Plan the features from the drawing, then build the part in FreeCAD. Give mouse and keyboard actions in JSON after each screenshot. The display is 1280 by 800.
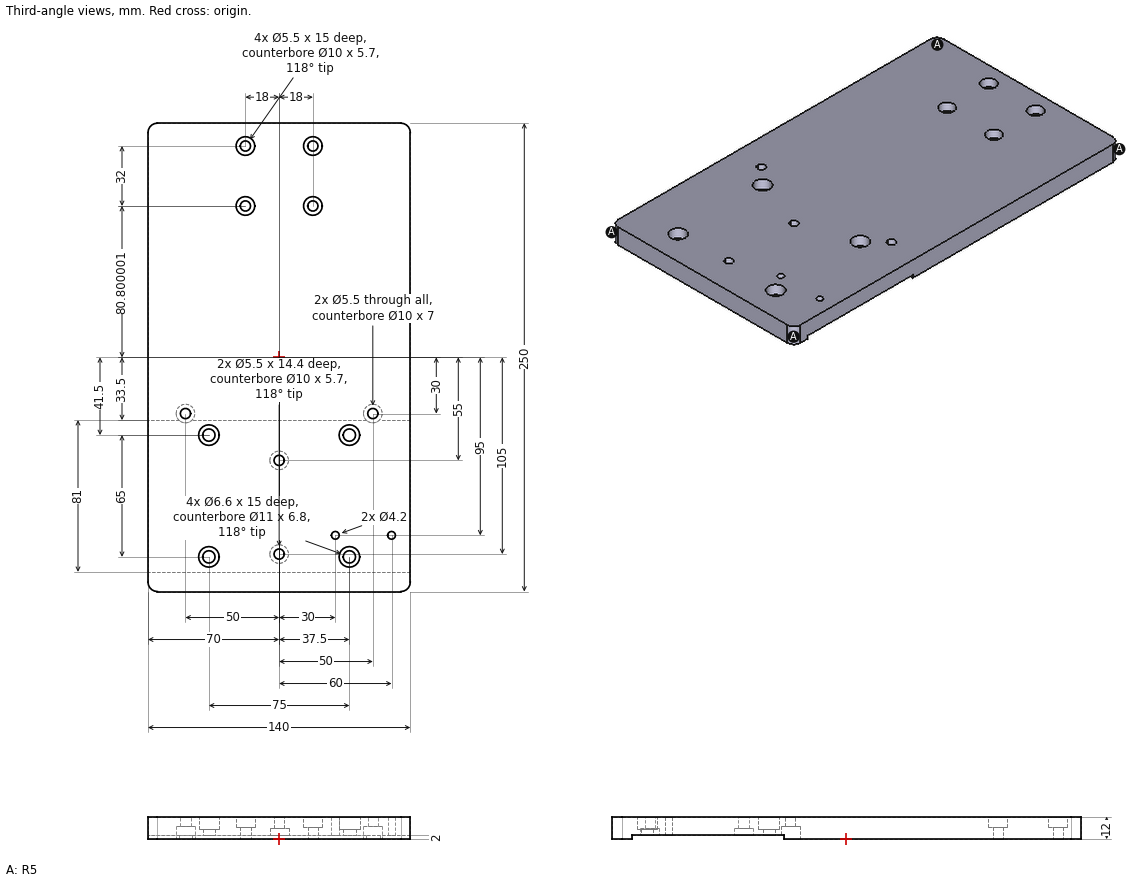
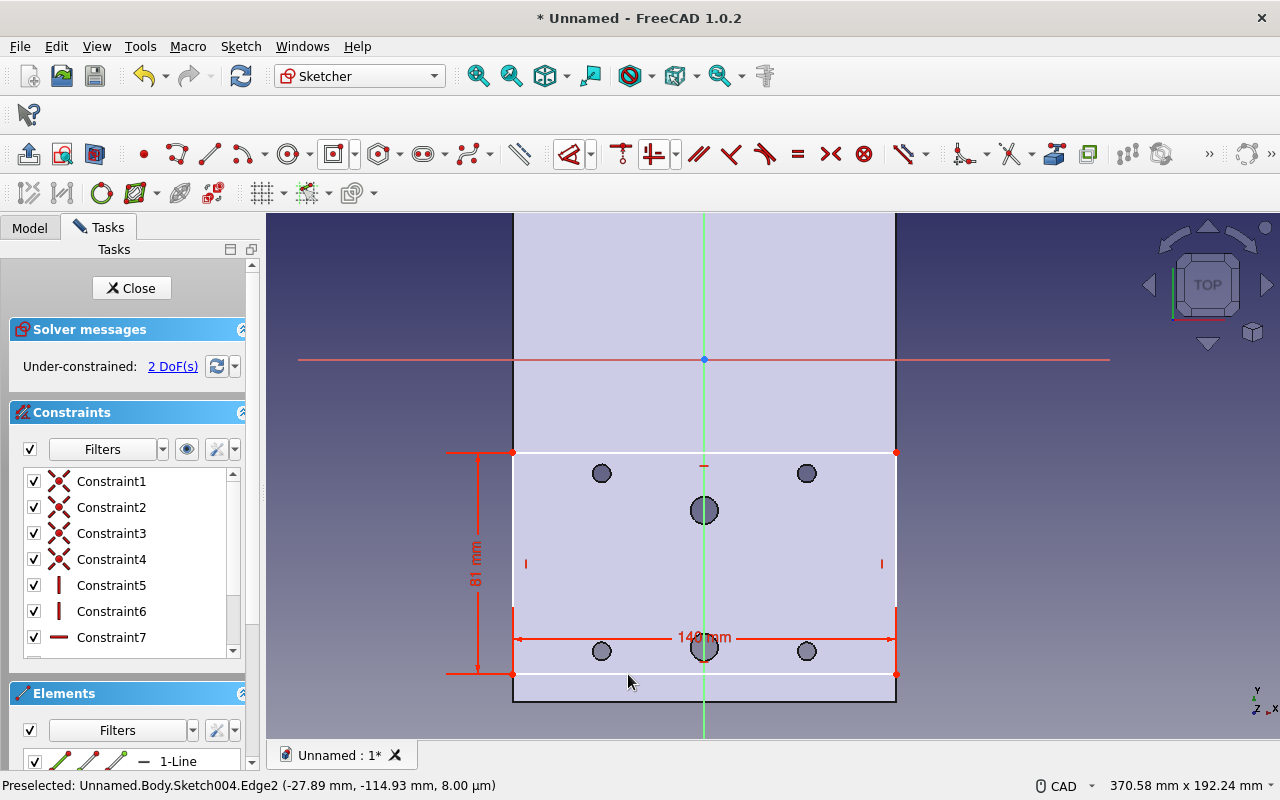
{"action": "left_click", "coordinate": [513, 453]}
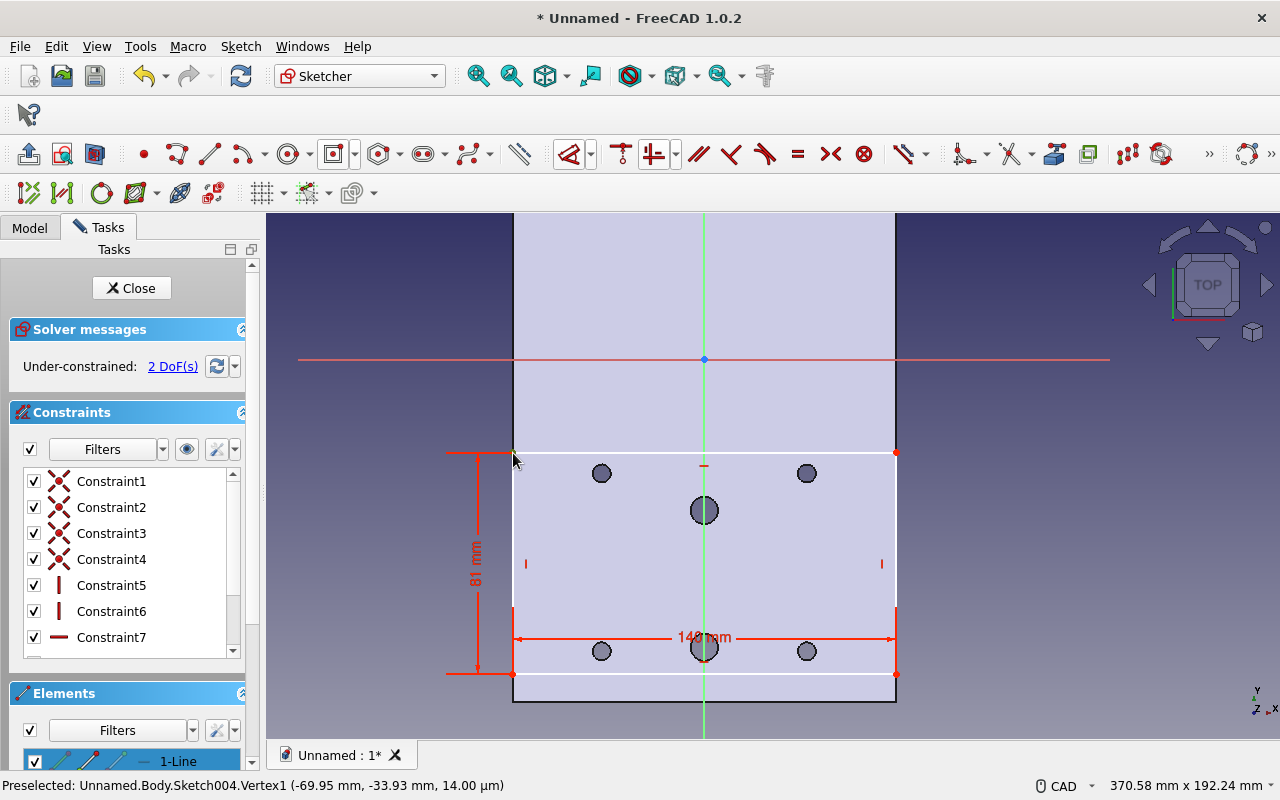
{"action": "left_click", "coordinate": [590, 154]}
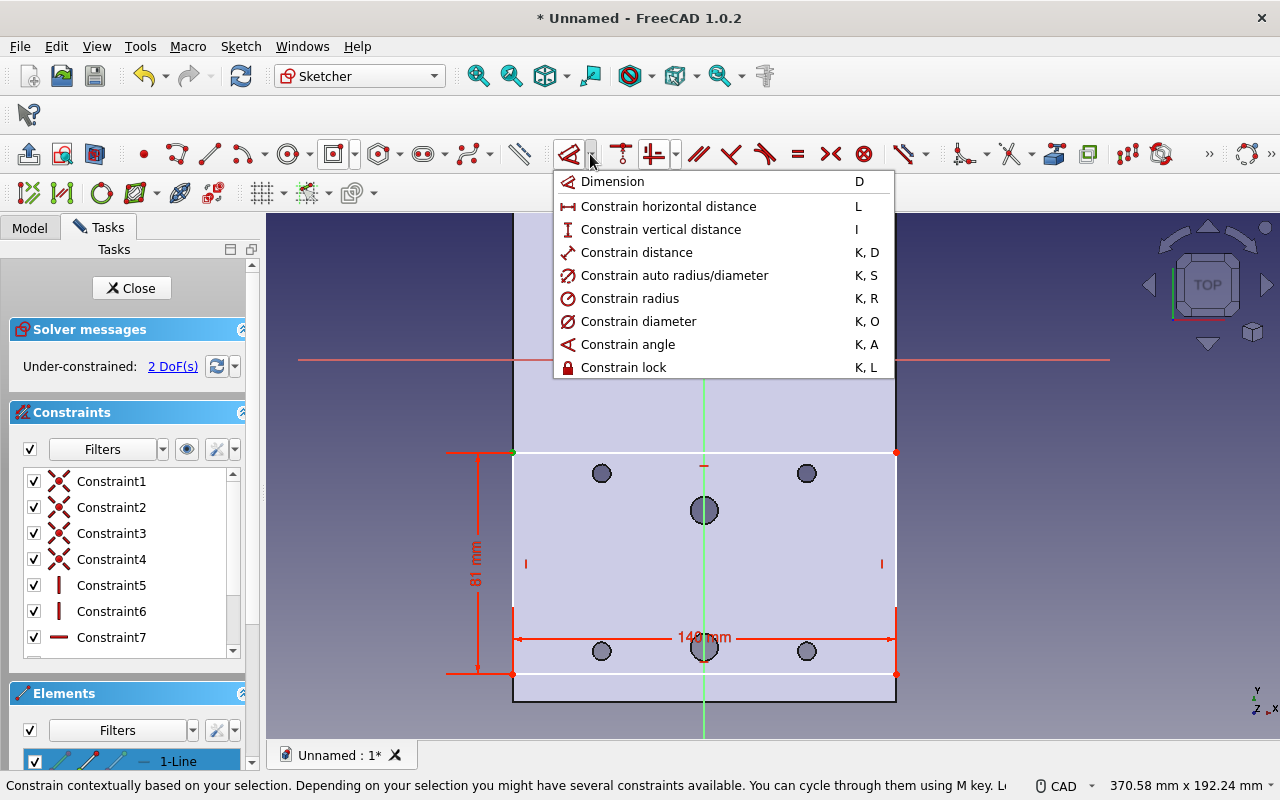
{"action": "left_click", "coordinate": [724, 206]}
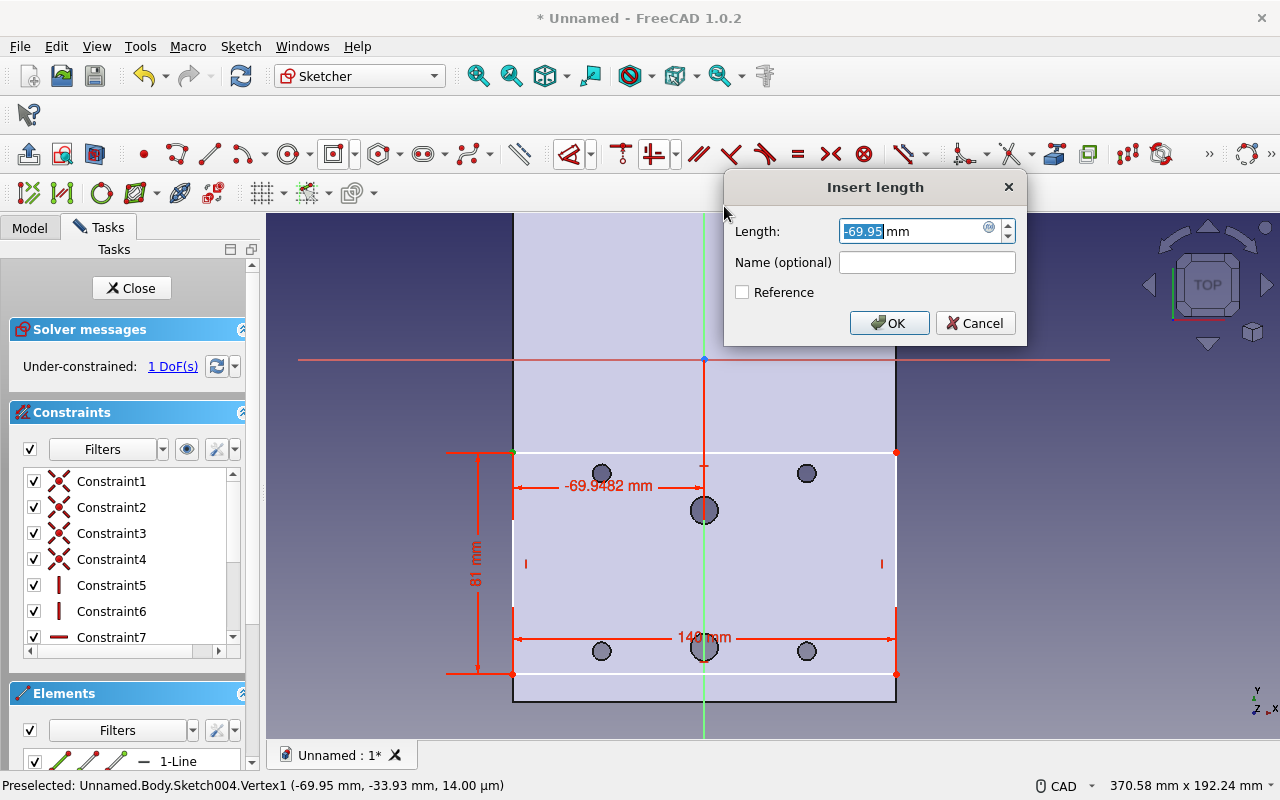
{"action": "type", "text": "-70"}
{"action": "key", "text": "Return"}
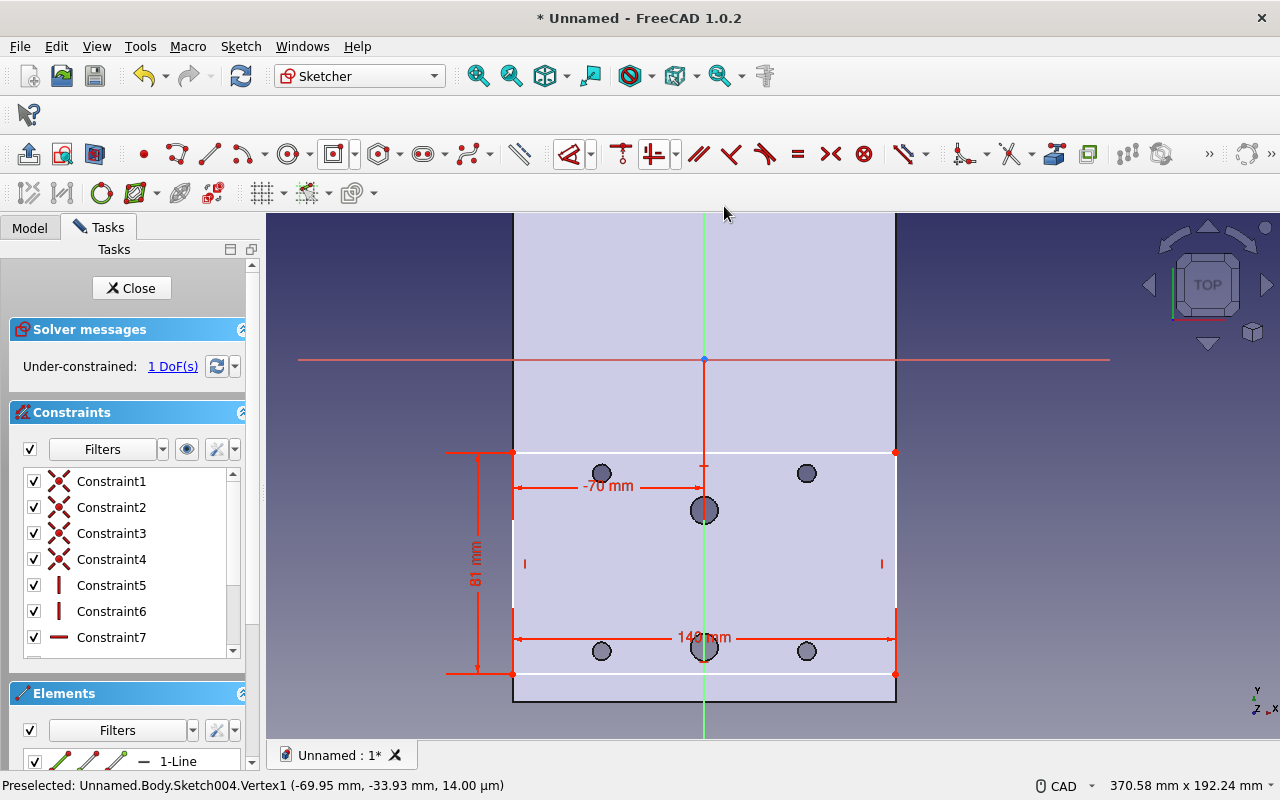
{"action": "left_click", "coordinate": [513, 453]}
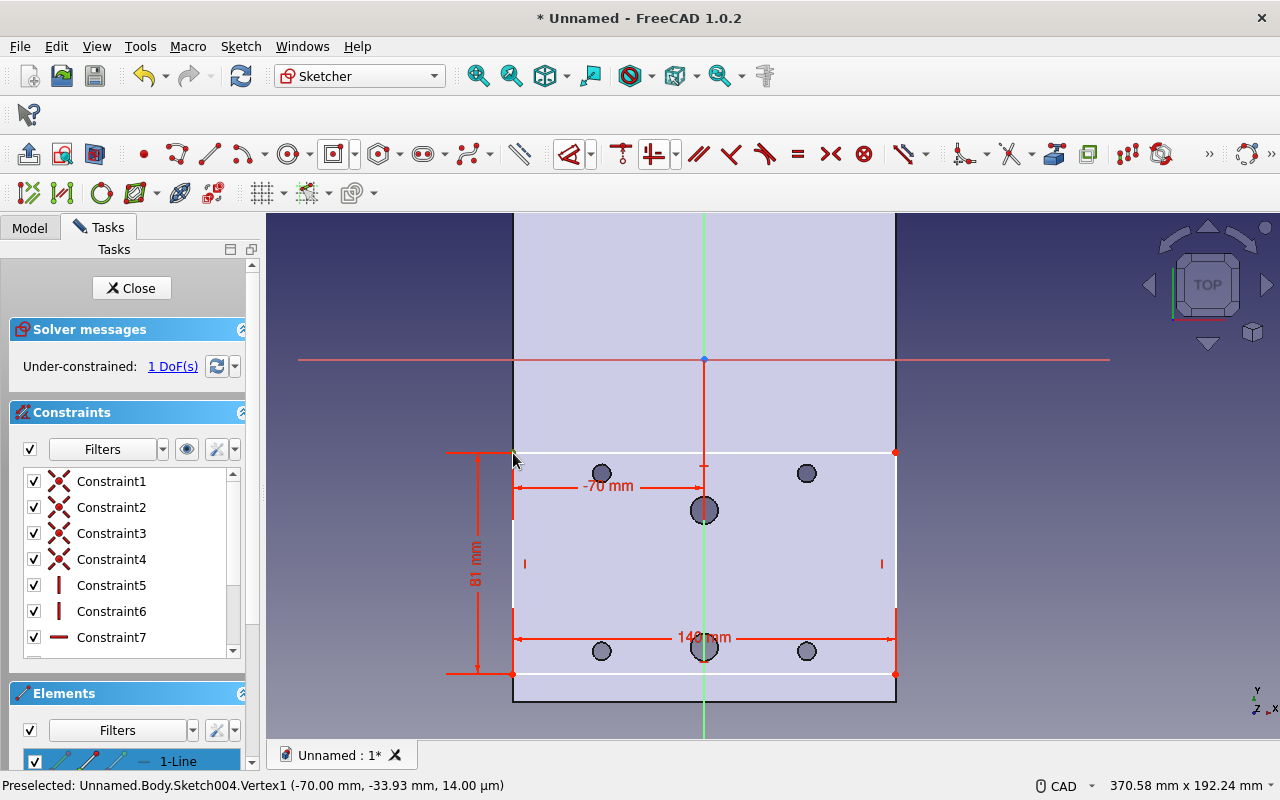
{"action": "left_click", "coordinate": [590, 154]}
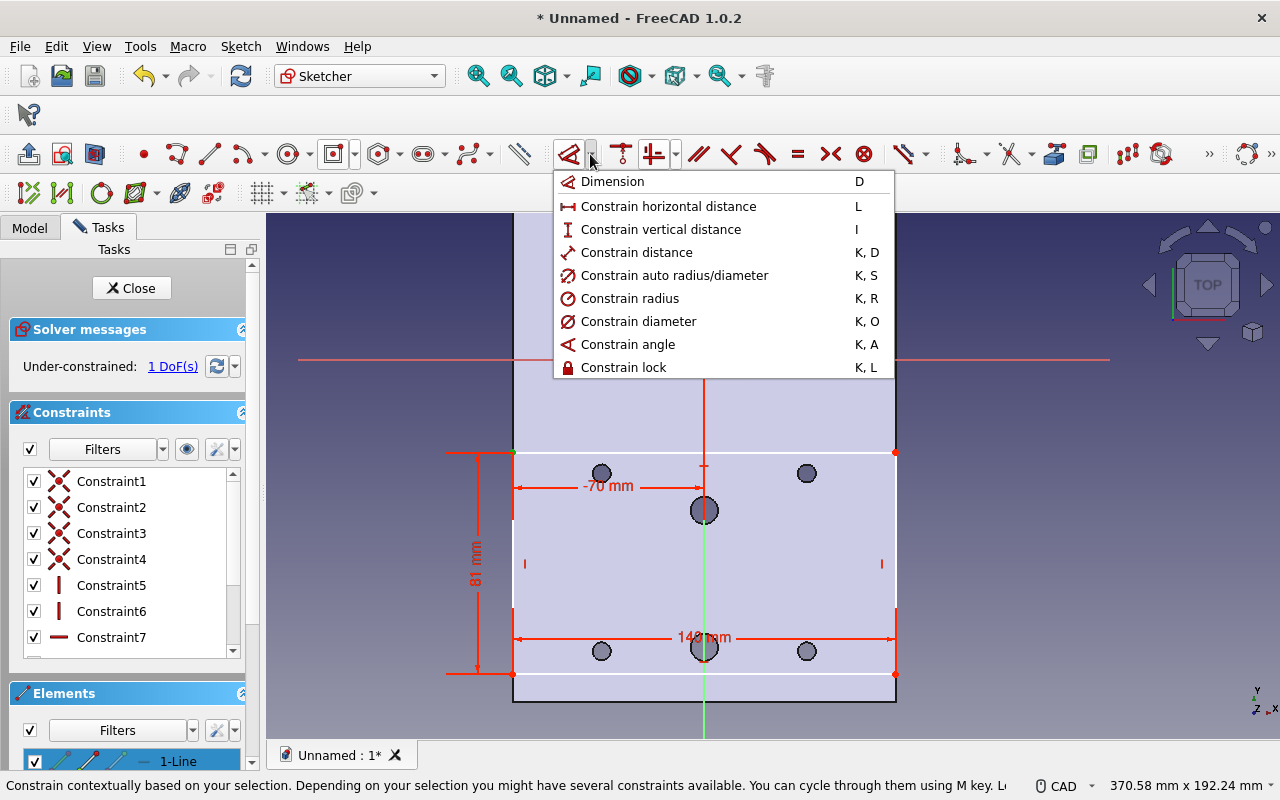
{"action": "left_click", "coordinate": [724, 230]}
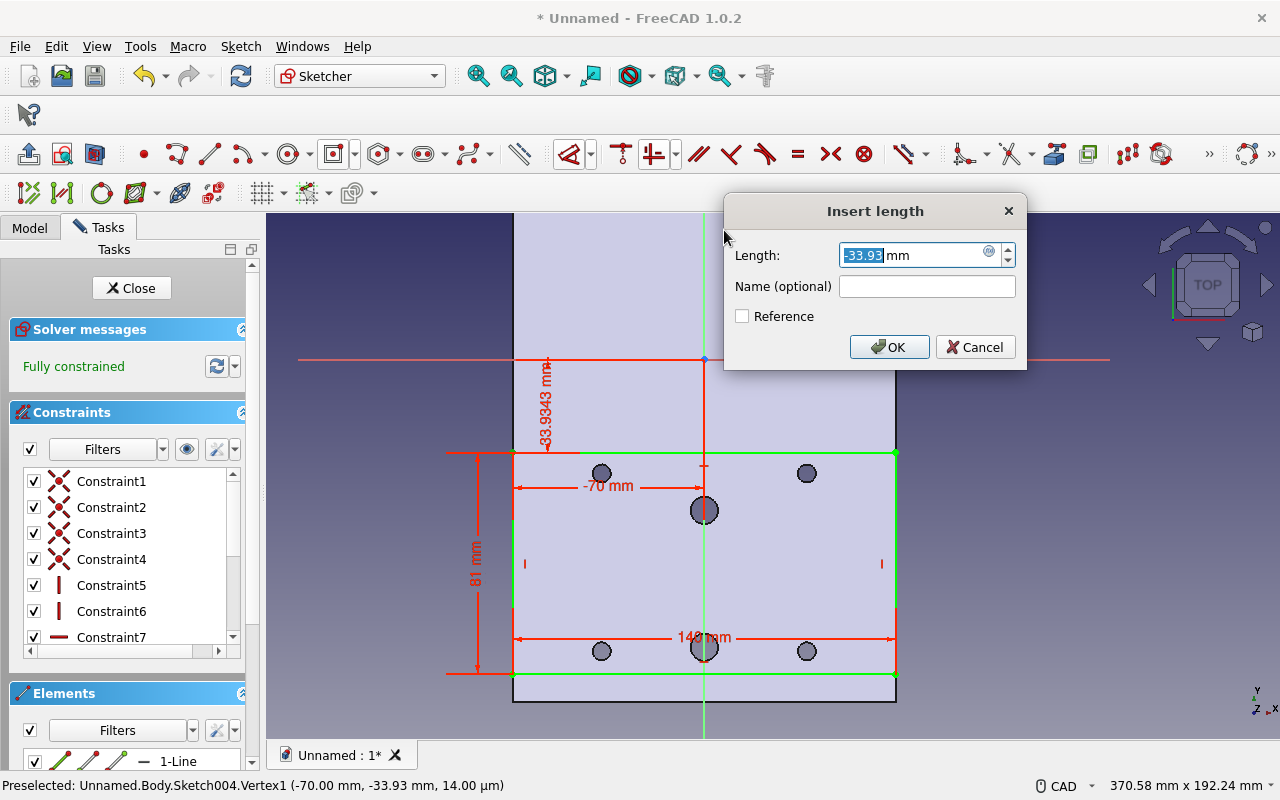
{"action": "type", "text": "-33.5"}
{"action": "key", "text": "Return"}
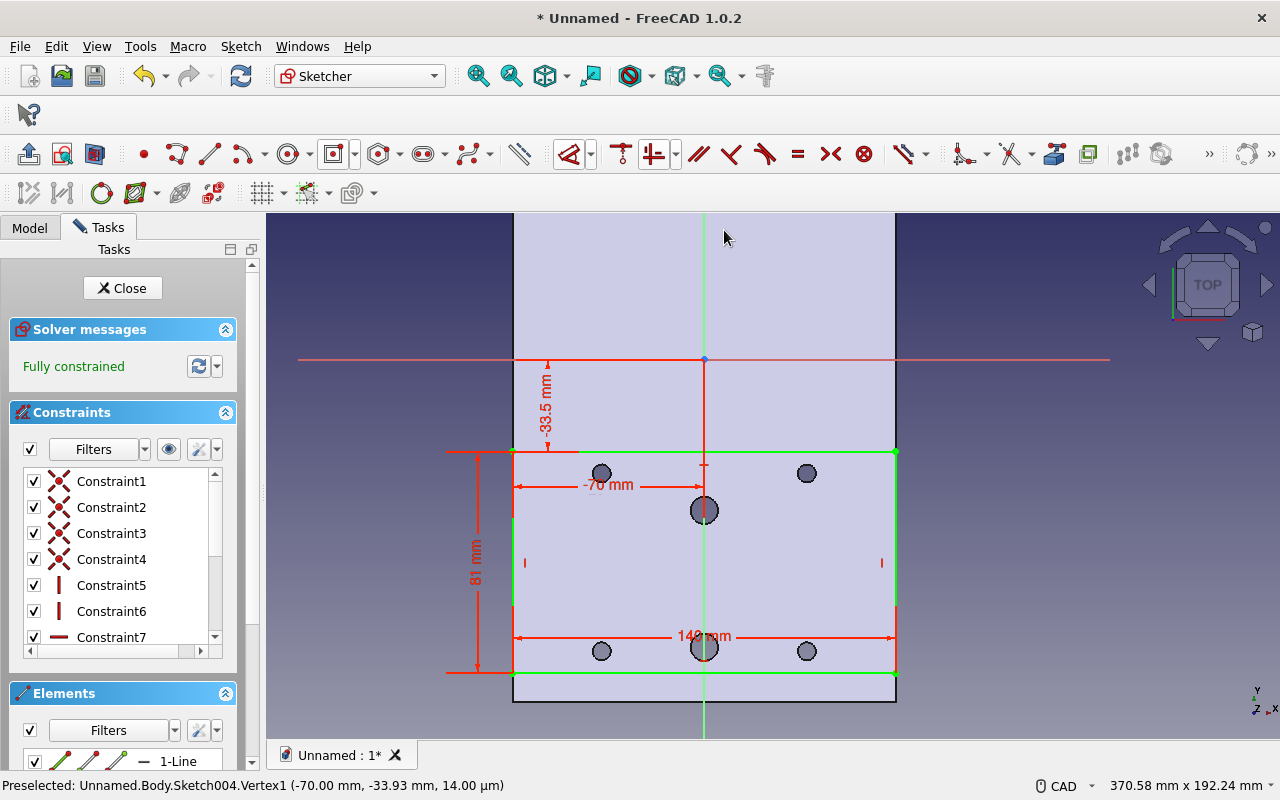
{"action": "left_click", "coordinate": [123, 288]}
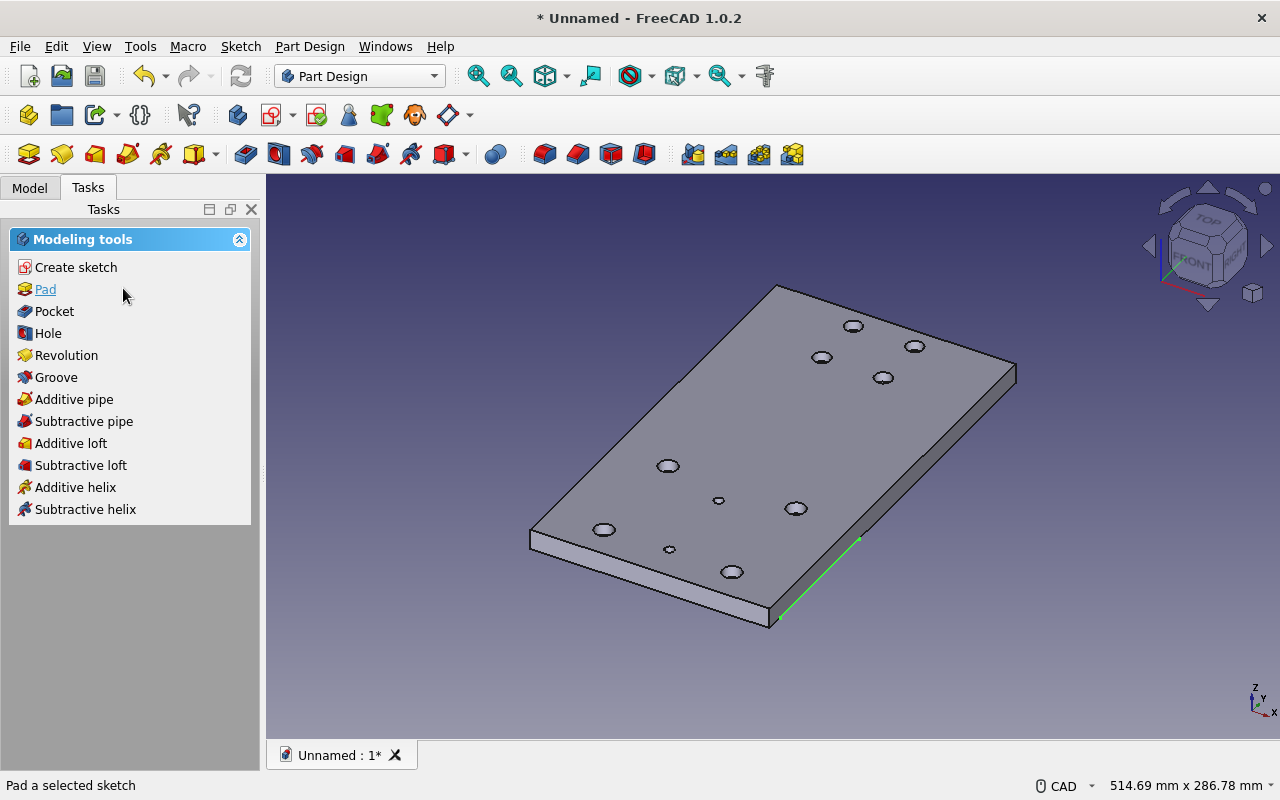
{"action": "left_click", "coordinate": [246, 154]}